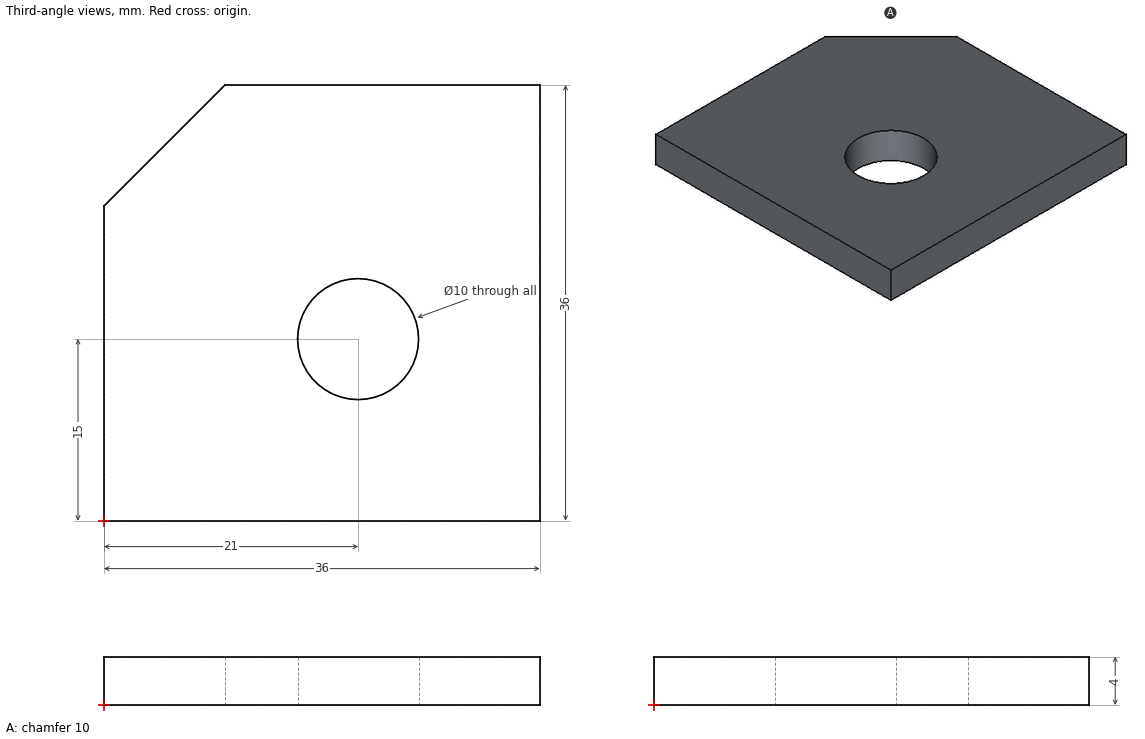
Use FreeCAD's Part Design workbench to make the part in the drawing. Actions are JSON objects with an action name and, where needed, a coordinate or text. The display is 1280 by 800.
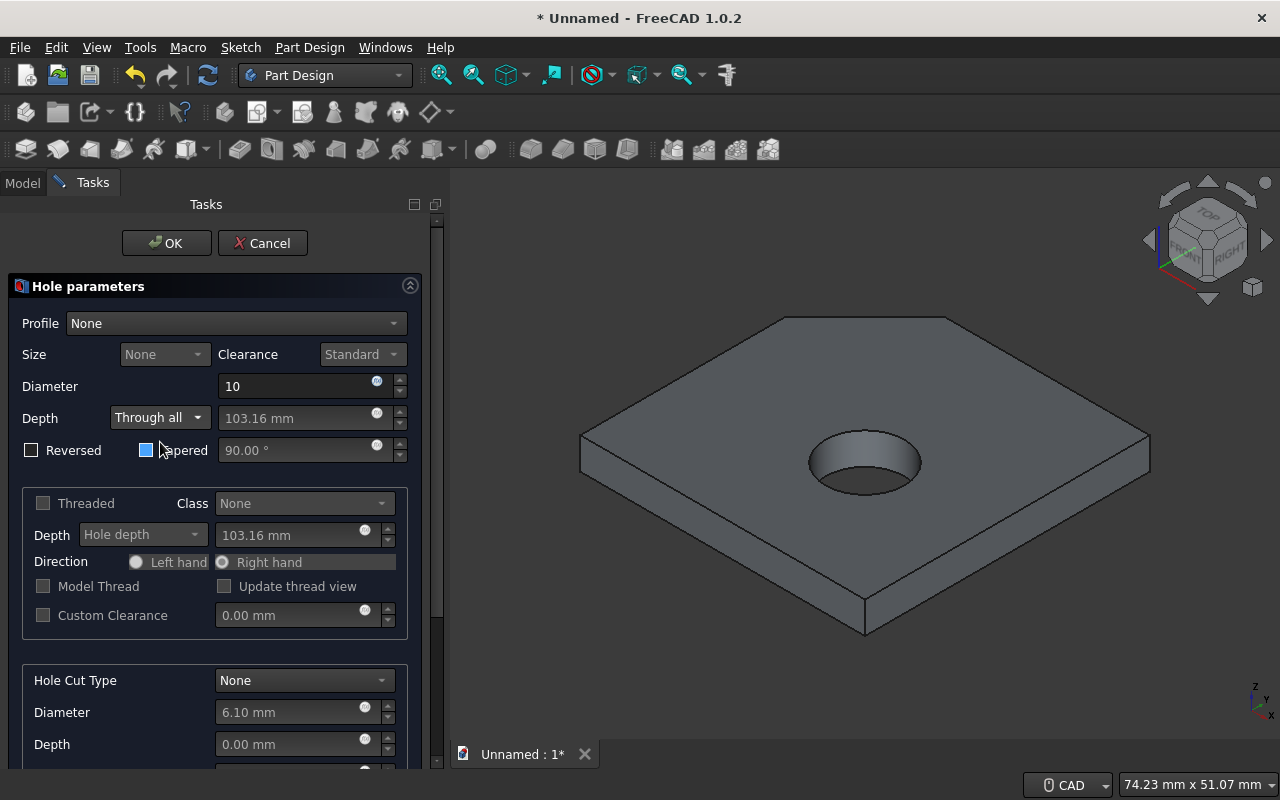
{"action": "left_click", "coordinate": [167, 243]}